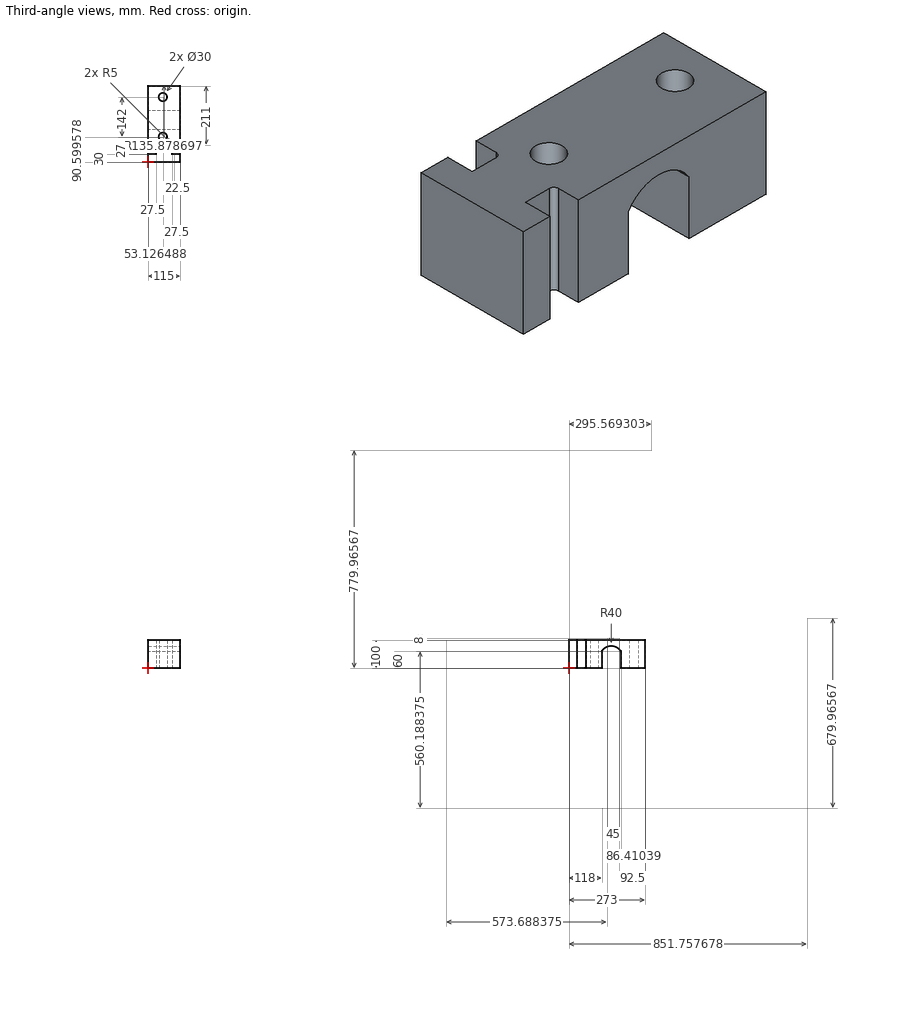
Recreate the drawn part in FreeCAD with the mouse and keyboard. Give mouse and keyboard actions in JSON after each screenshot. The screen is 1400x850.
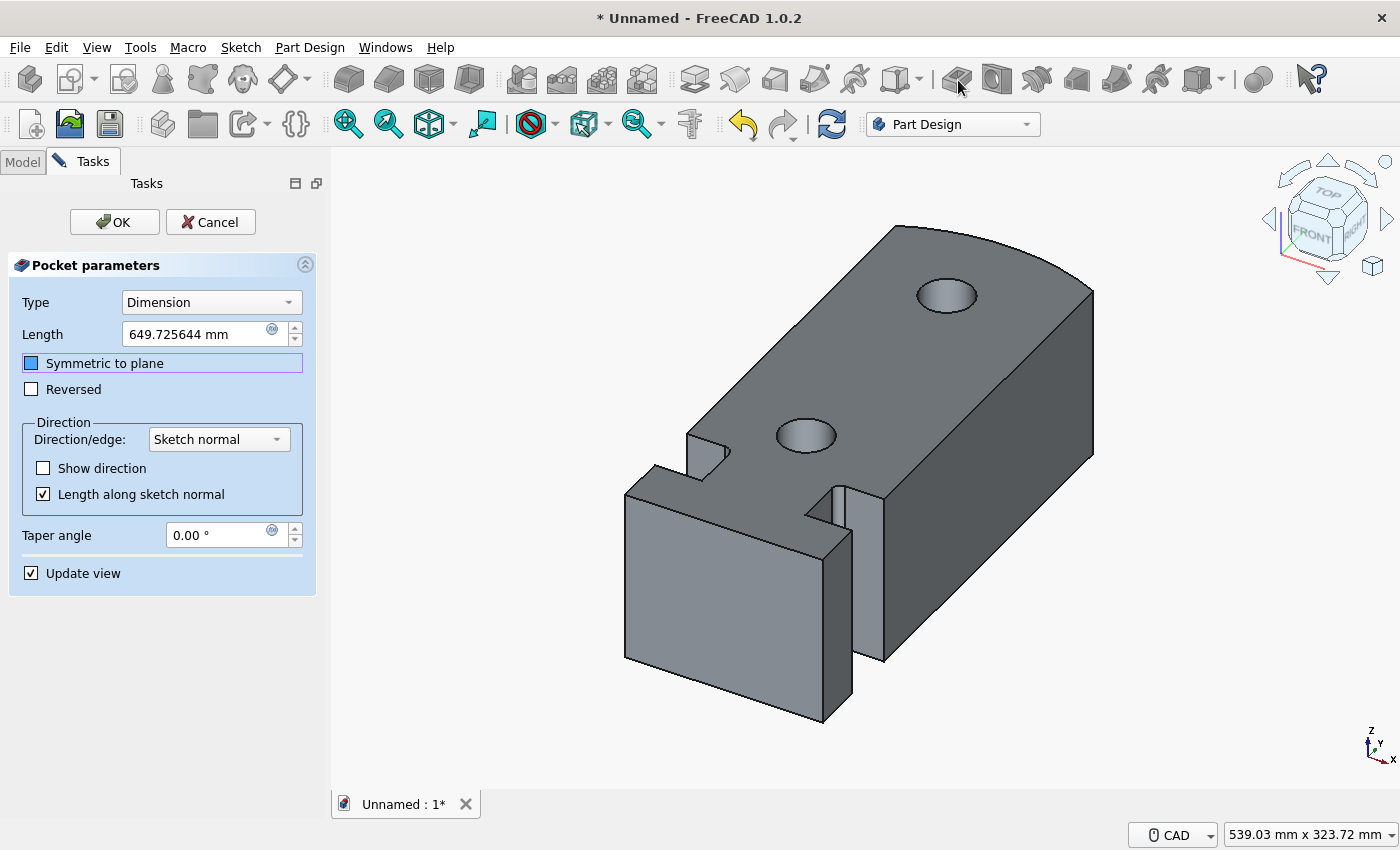
{"action": "left_click", "coordinate": [30, 363]}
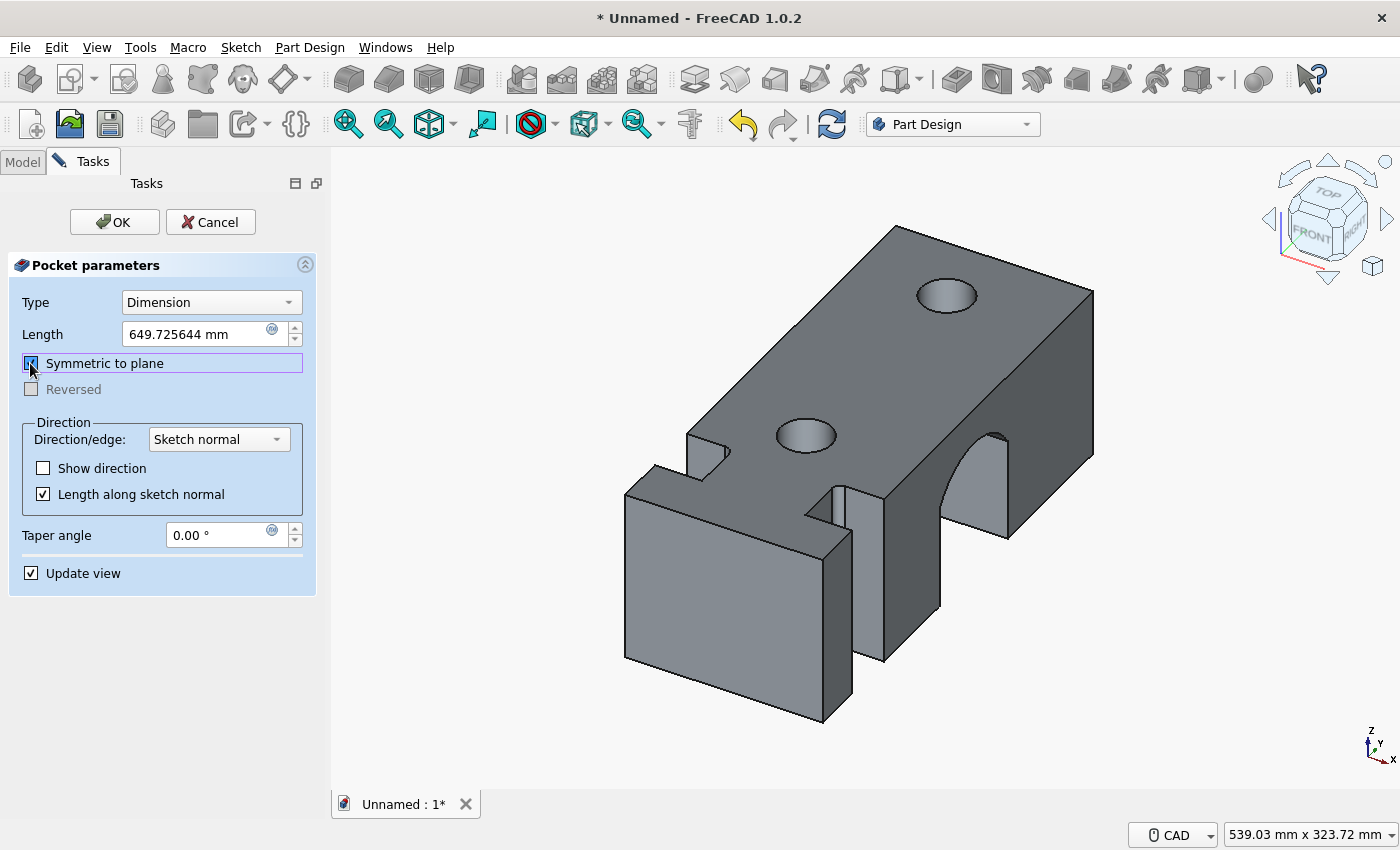
{"action": "left_click", "coordinate": [115, 222]}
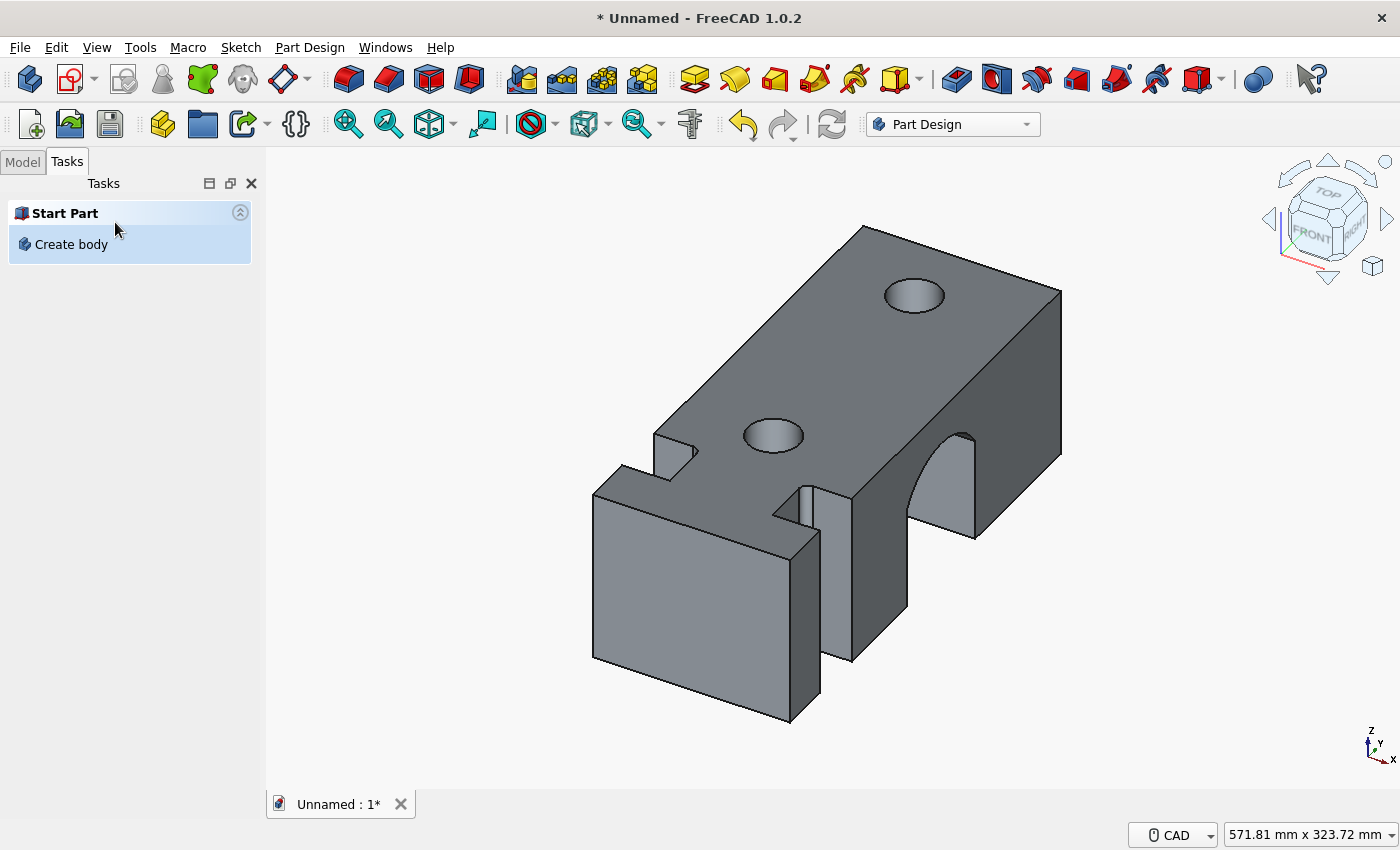
{"action": "key", "text": "0"}